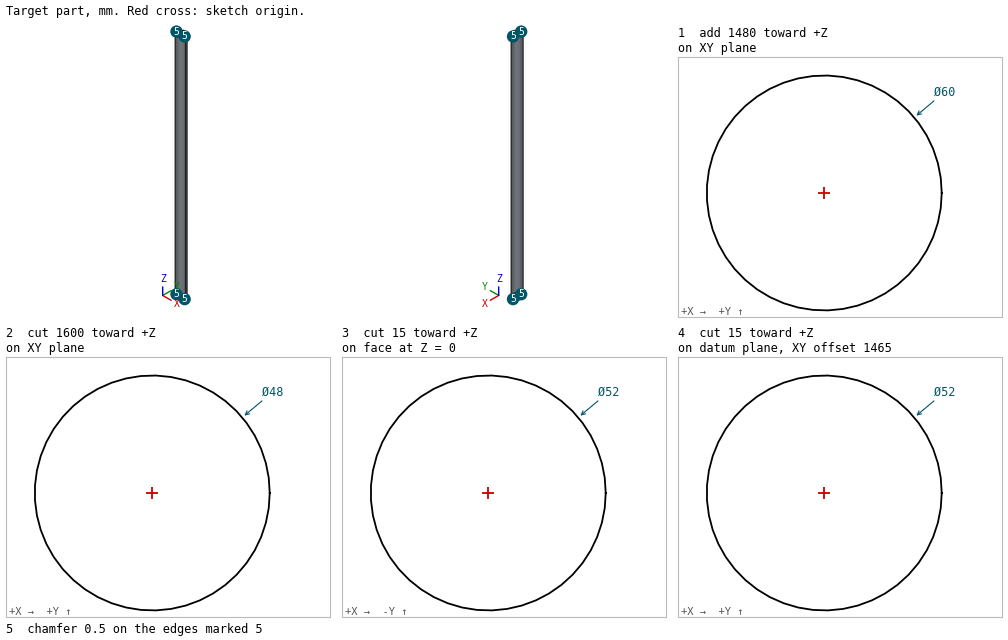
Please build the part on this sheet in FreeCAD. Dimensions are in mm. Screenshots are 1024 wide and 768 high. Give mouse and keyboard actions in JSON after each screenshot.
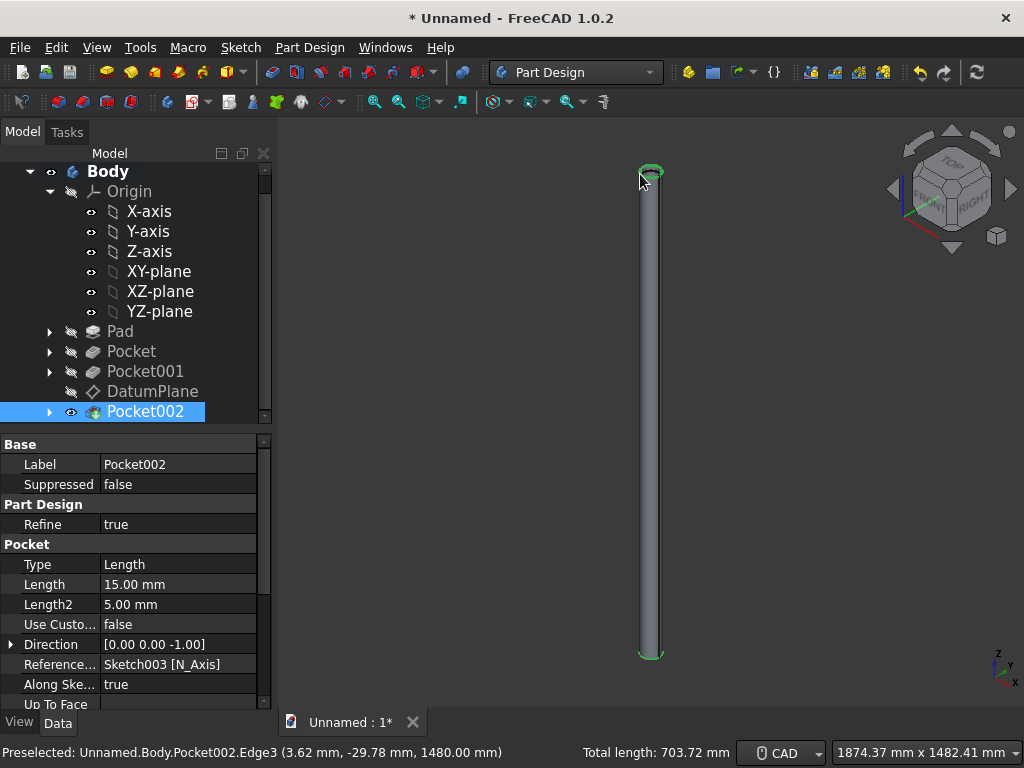
{"action": "left_click", "coordinate": [84, 102]}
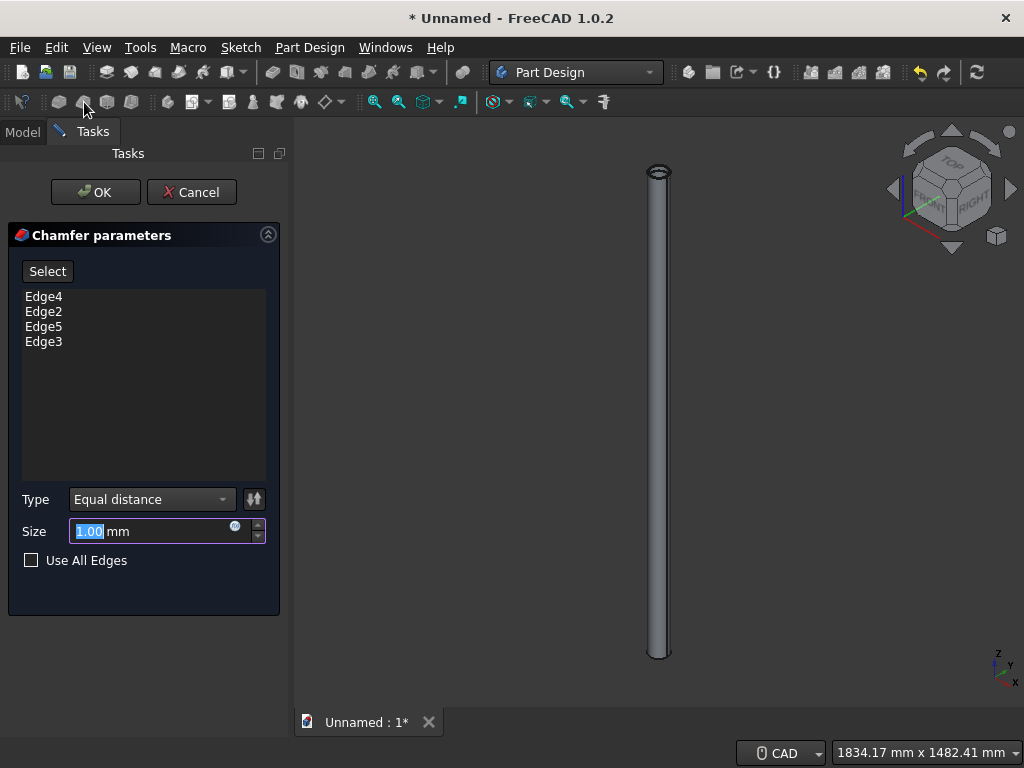
{"action": "type", "text": "0.5"}
{"action": "key", "text": "Tab"}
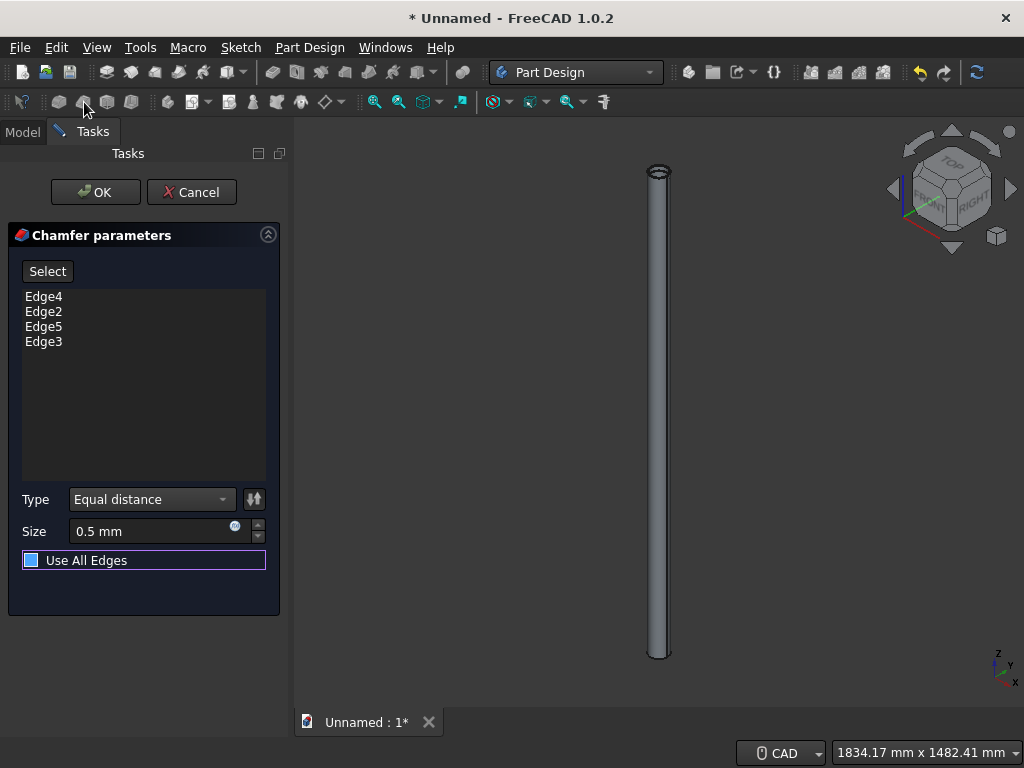
{"action": "left_click", "coordinate": [96, 192]}